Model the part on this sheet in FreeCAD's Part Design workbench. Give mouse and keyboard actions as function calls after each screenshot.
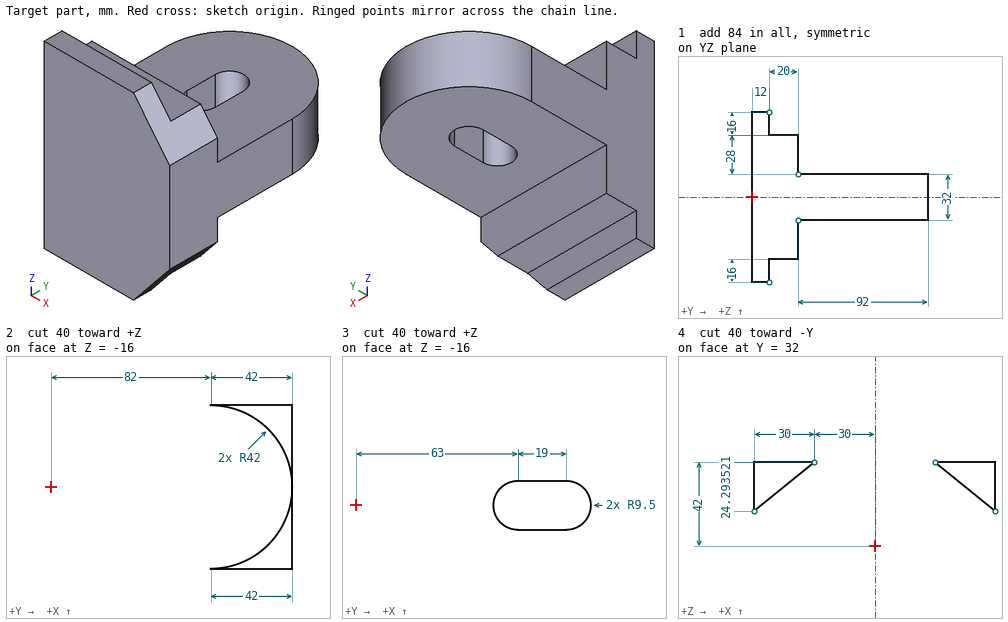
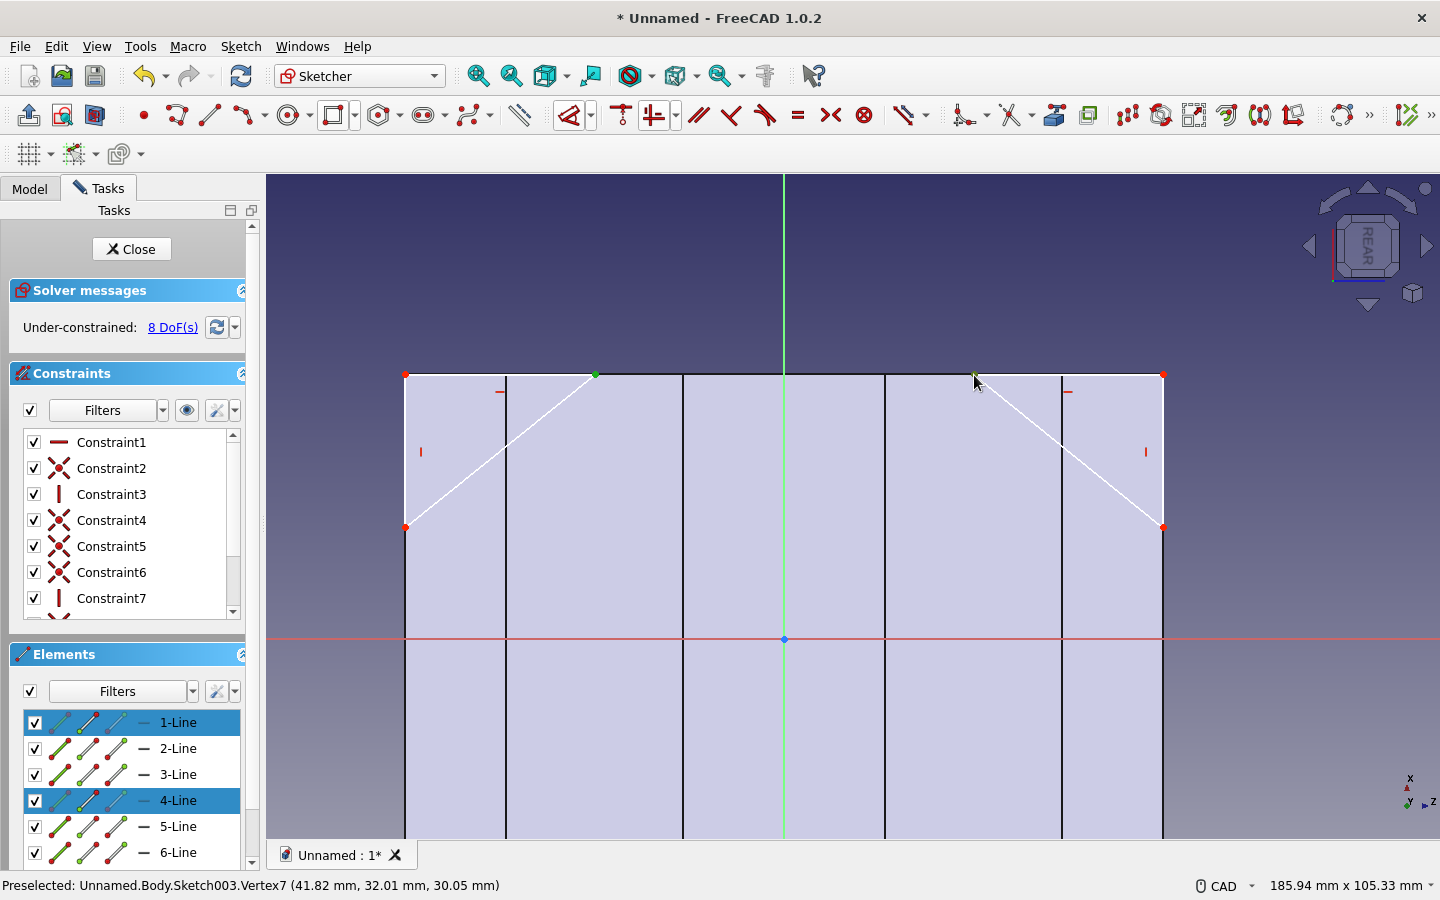
click(784, 768)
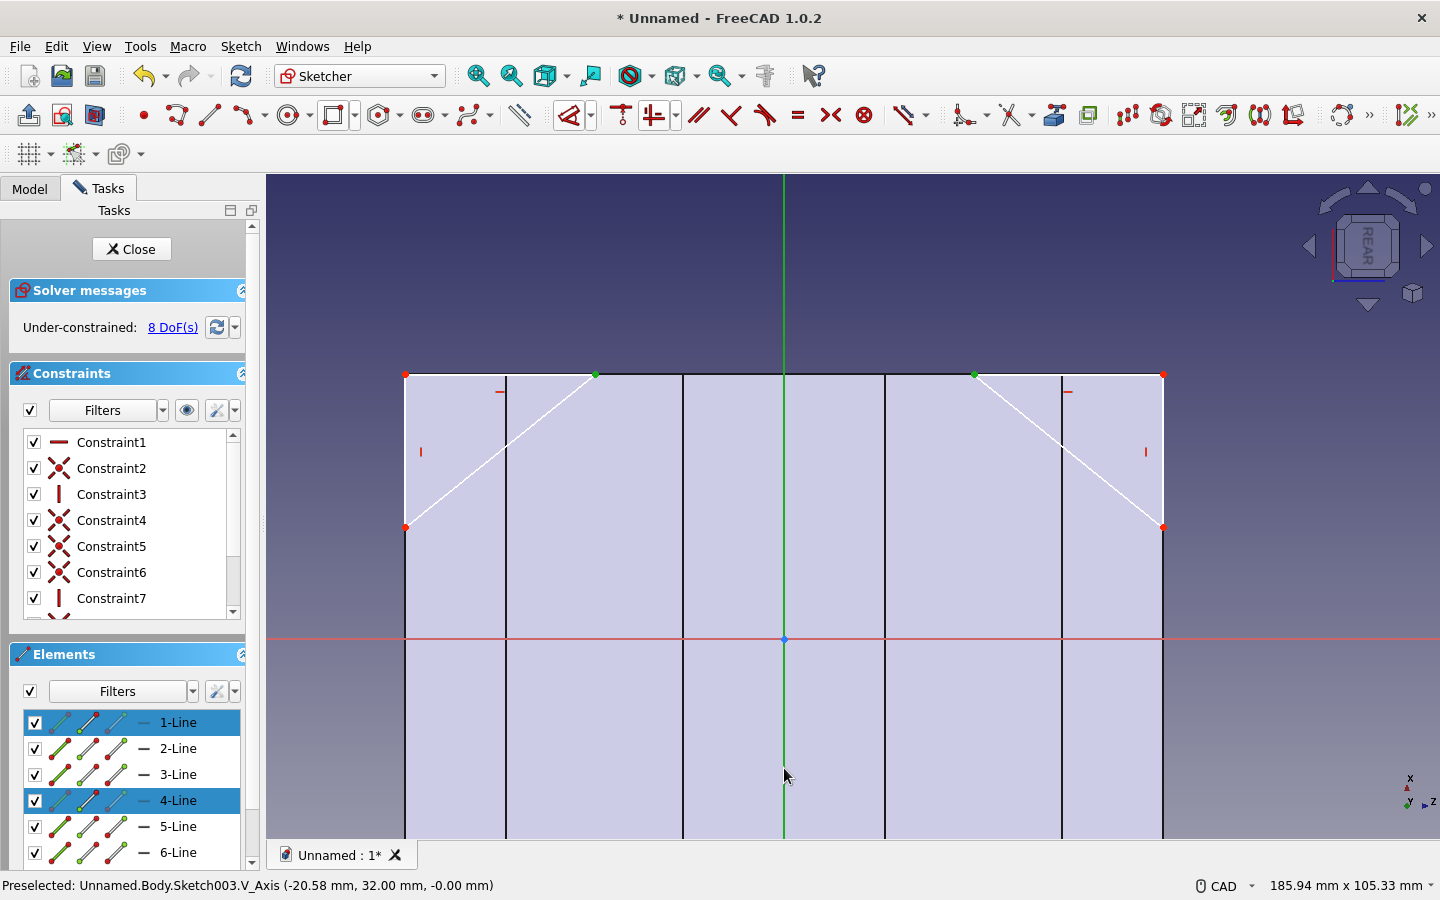
click(831, 116)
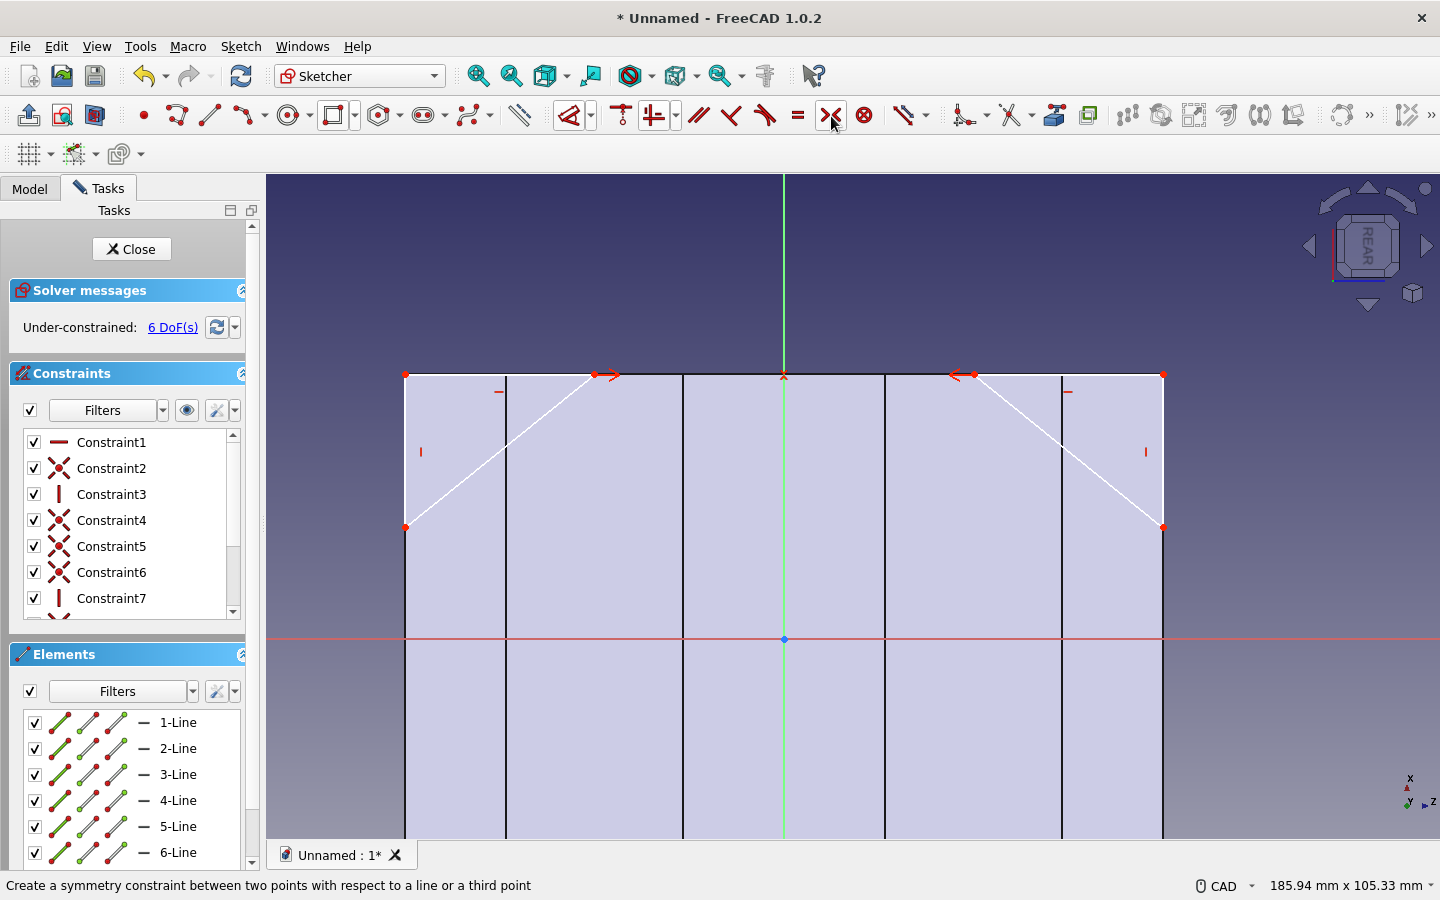
click(405, 528)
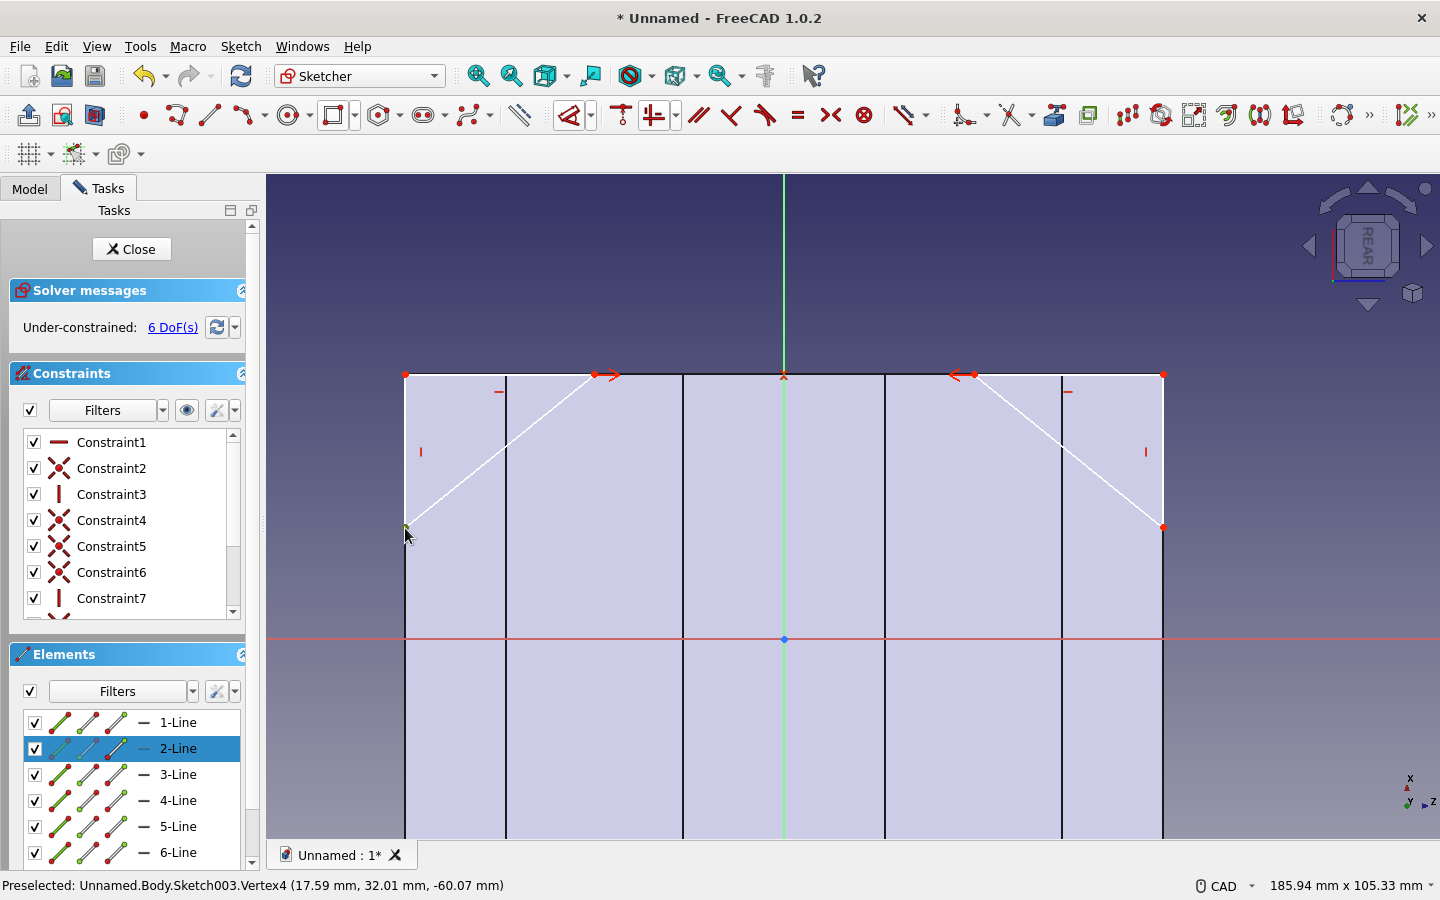
click(1163, 528)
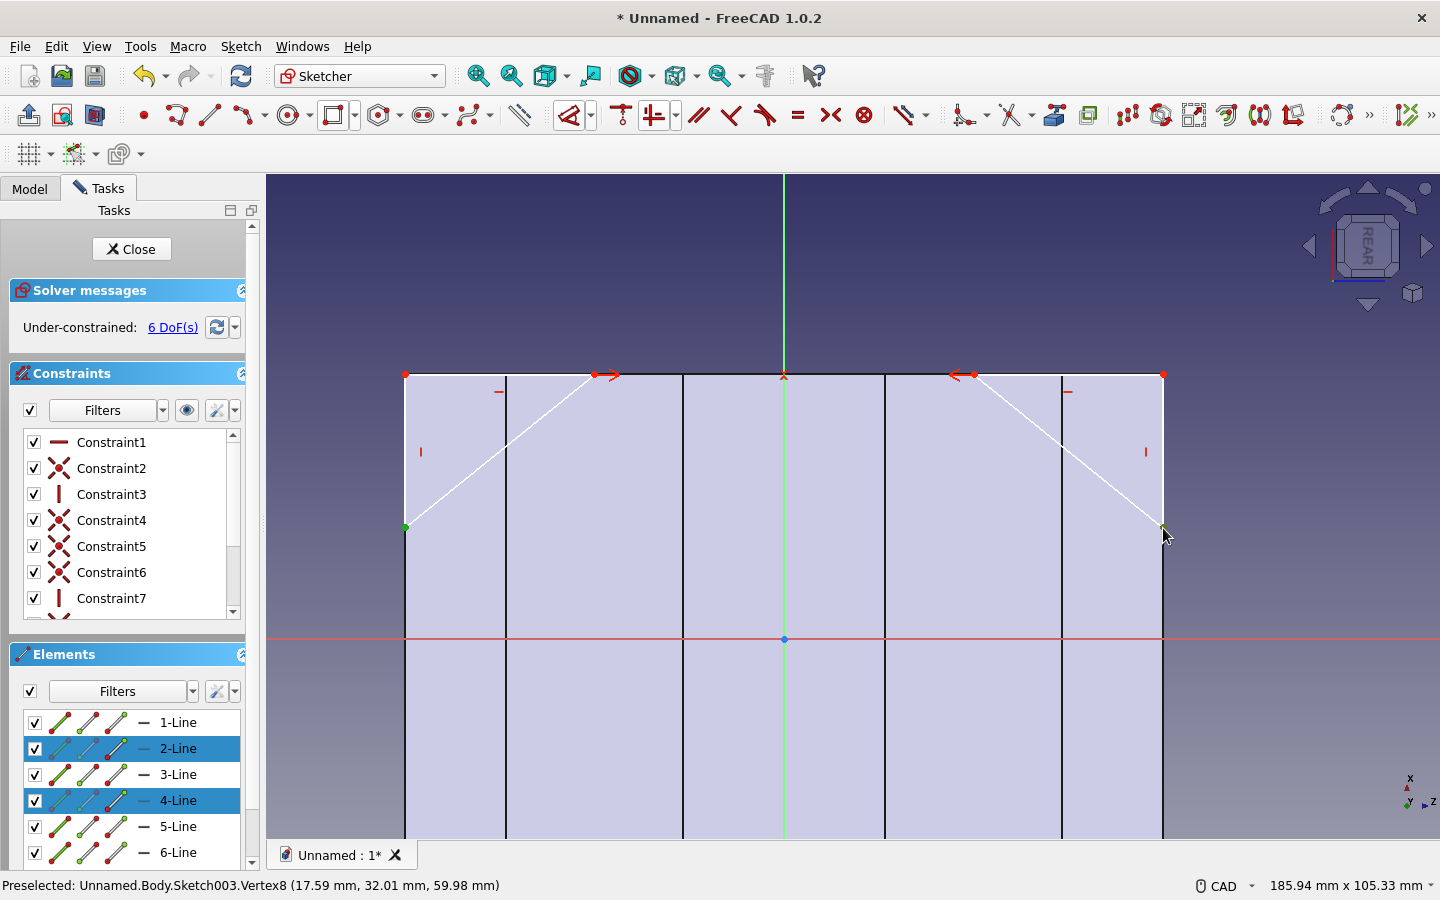
click(784, 768)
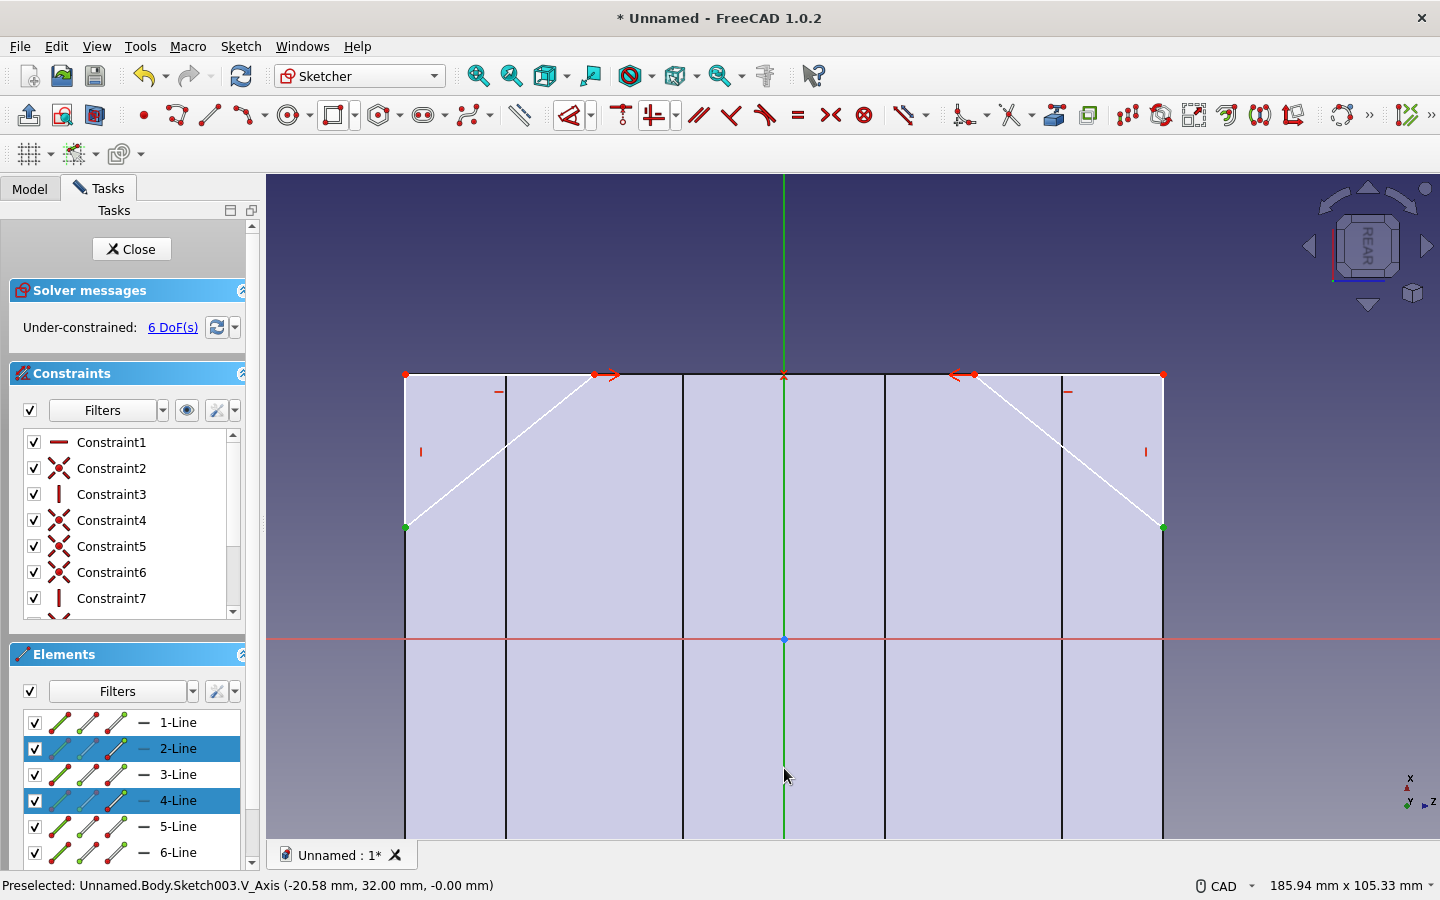
click(831, 116)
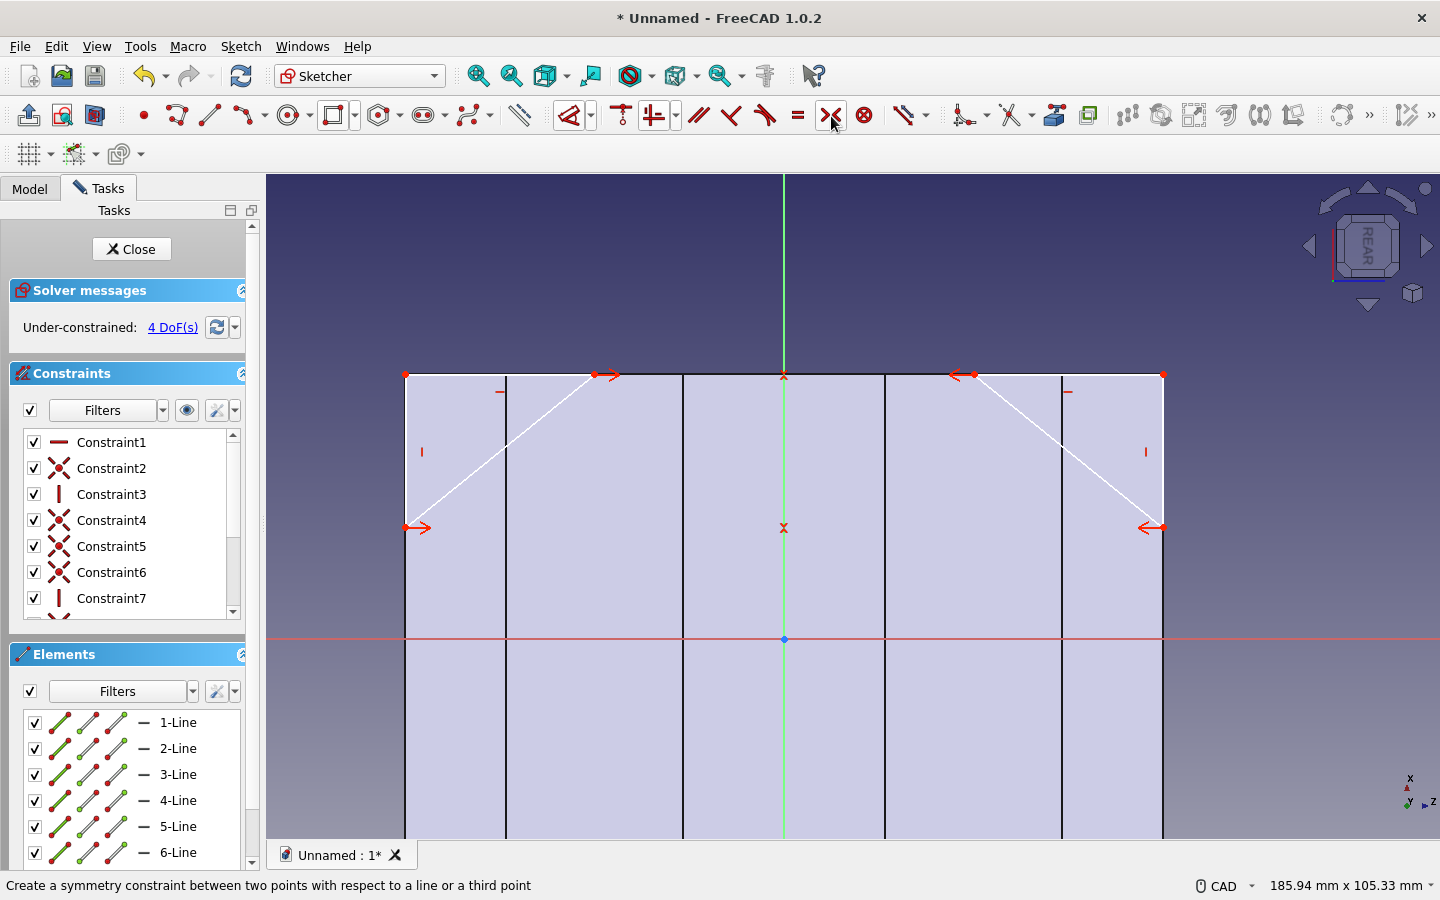
click(538, 375)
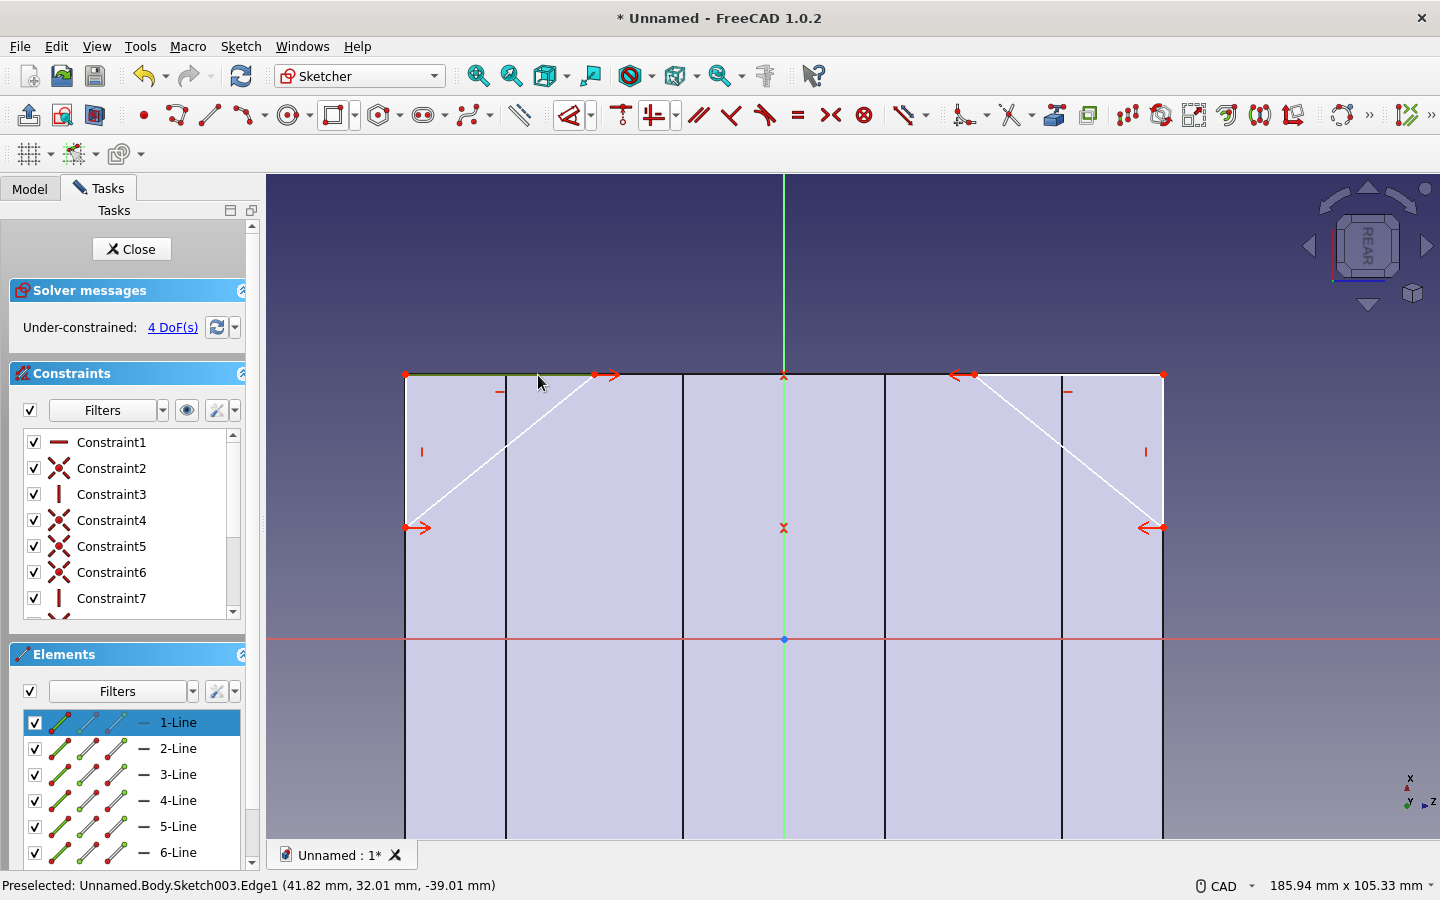
key(l)